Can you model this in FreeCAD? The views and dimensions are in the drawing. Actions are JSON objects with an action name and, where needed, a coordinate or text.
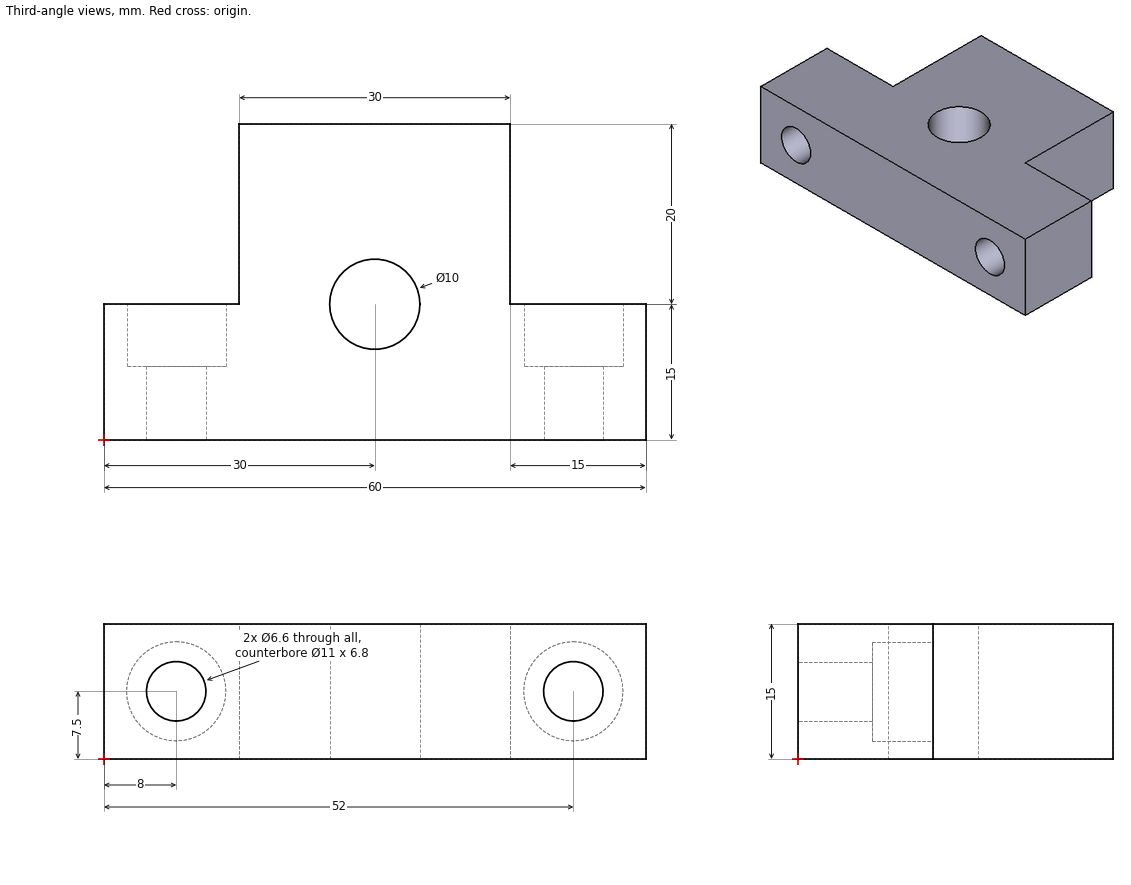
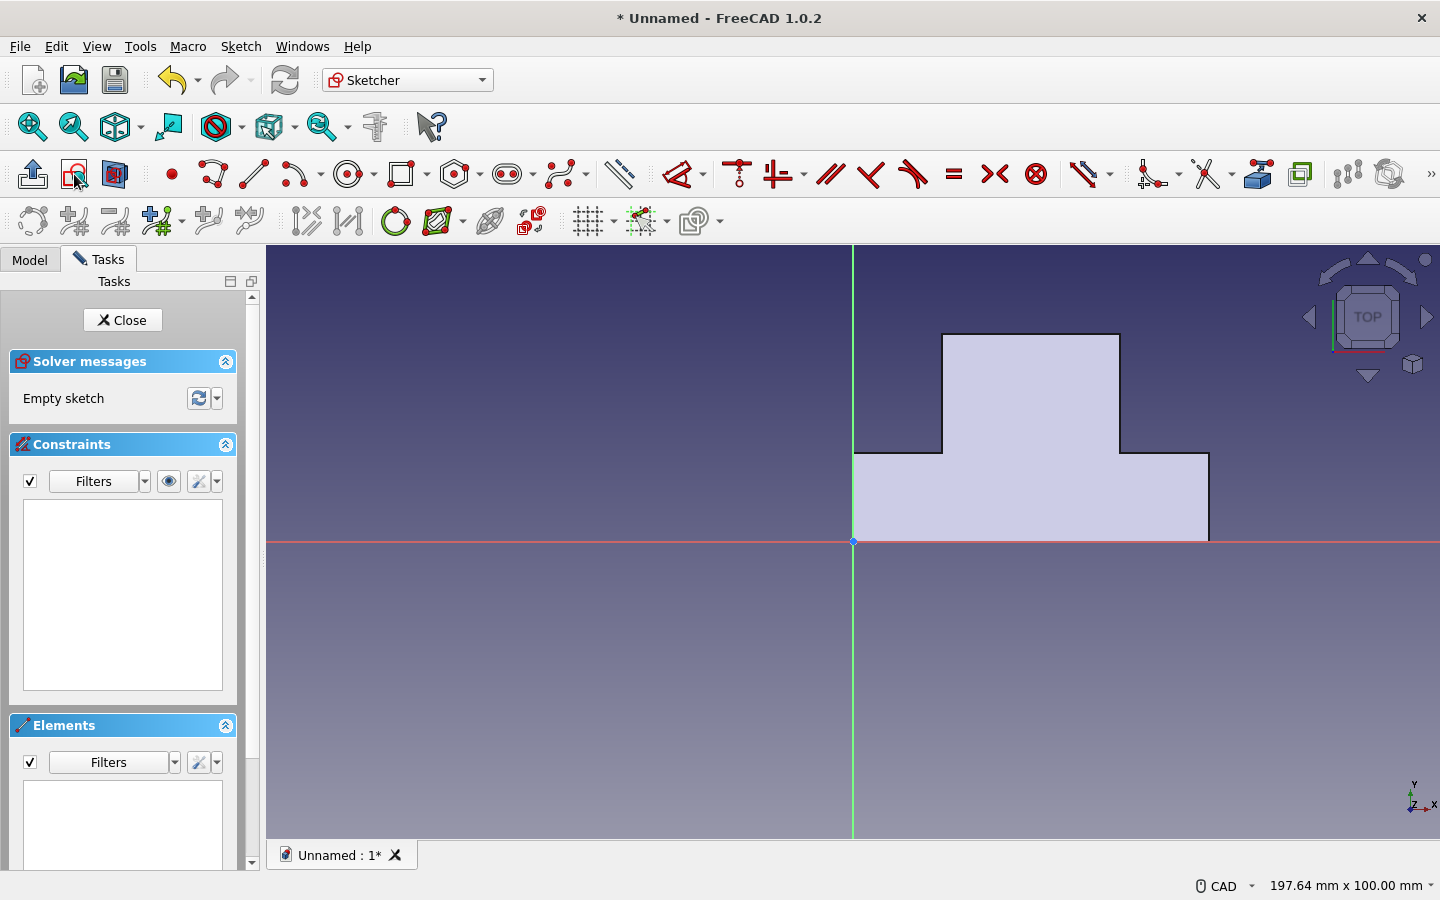
{"action": "scroll", "coordinate": [1080, 435], "scroll_direction": "up", "scroll_amount": 9}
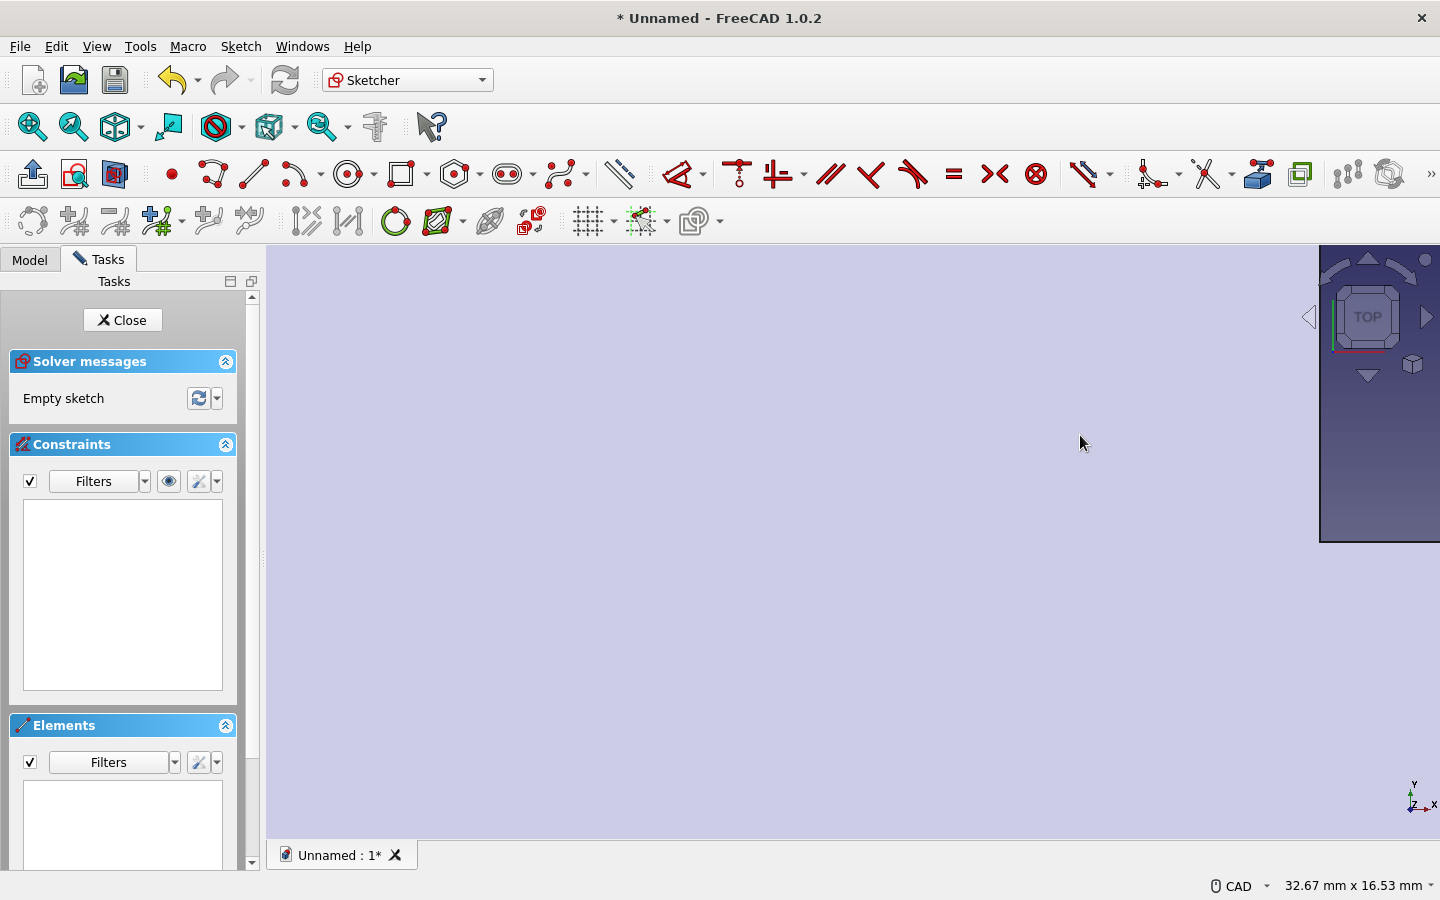
{"action": "left_click", "coordinate": [348, 174]}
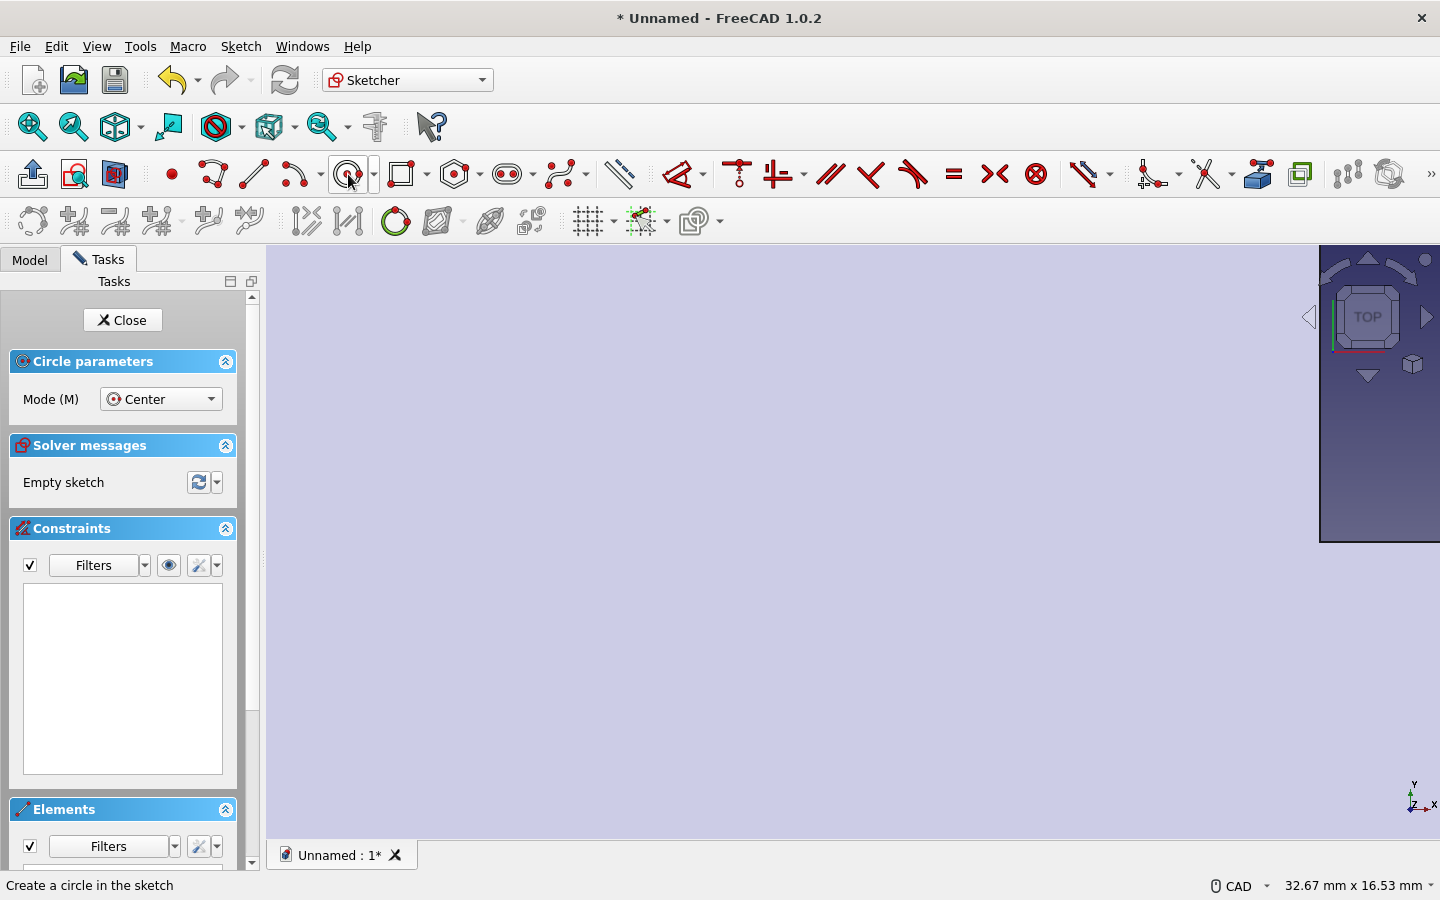
{"action": "left_click", "coordinate": [781, 542]}
{"action": "left_click", "coordinate": [908, 415]}
{"action": "key", "text": "Escape"}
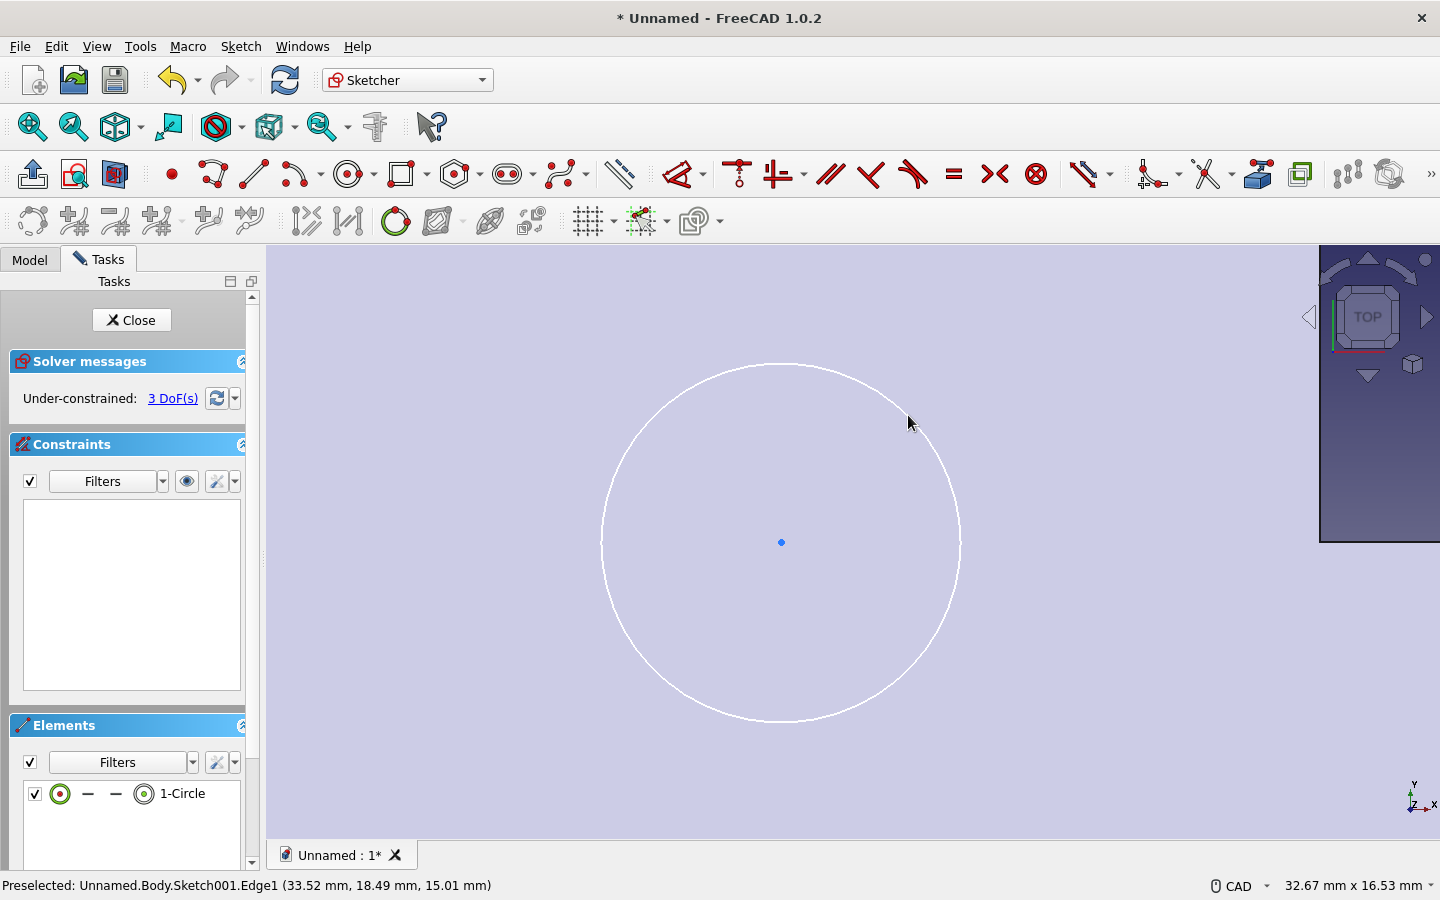
{"action": "left_click", "coordinate": [676, 174]}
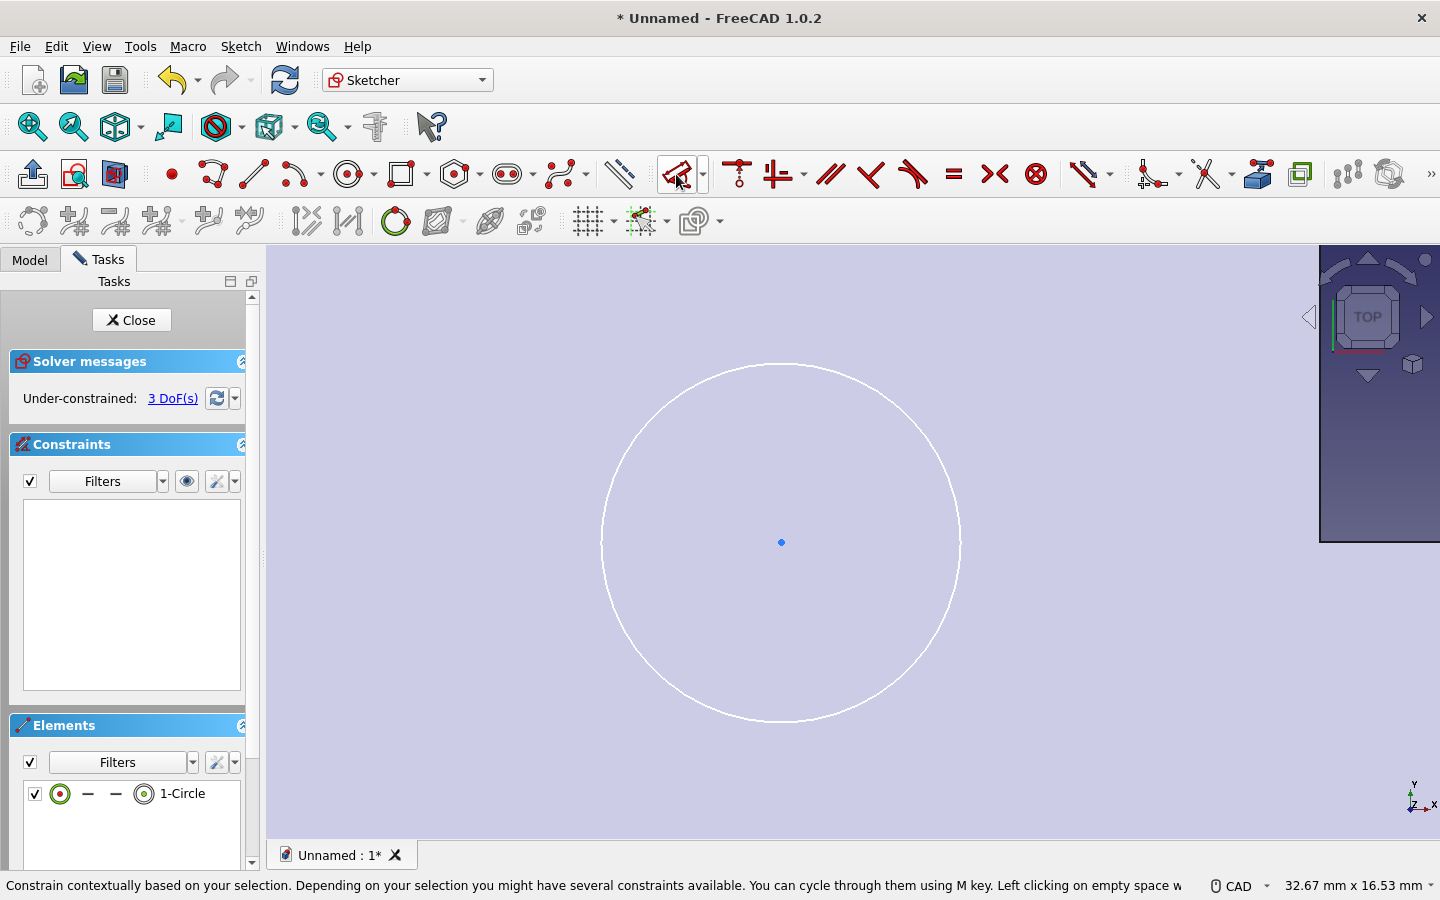
{"action": "left_click", "coordinate": [908, 416]}
{"action": "left_click", "coordinate": [931, 393]}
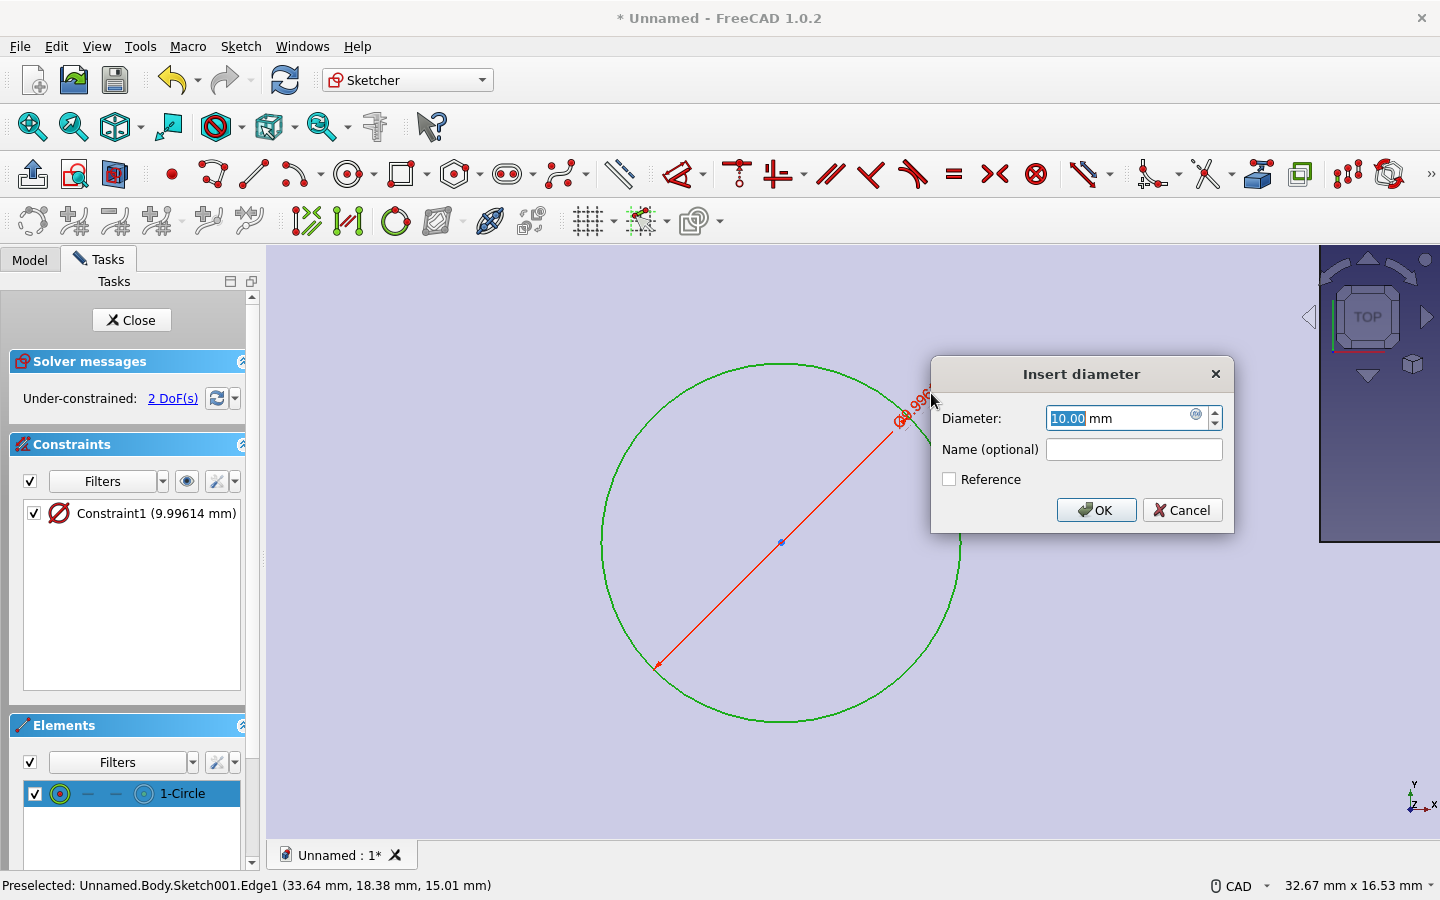
{"action": "type", "text": "10"}
{"action": "key", "text": "Return"}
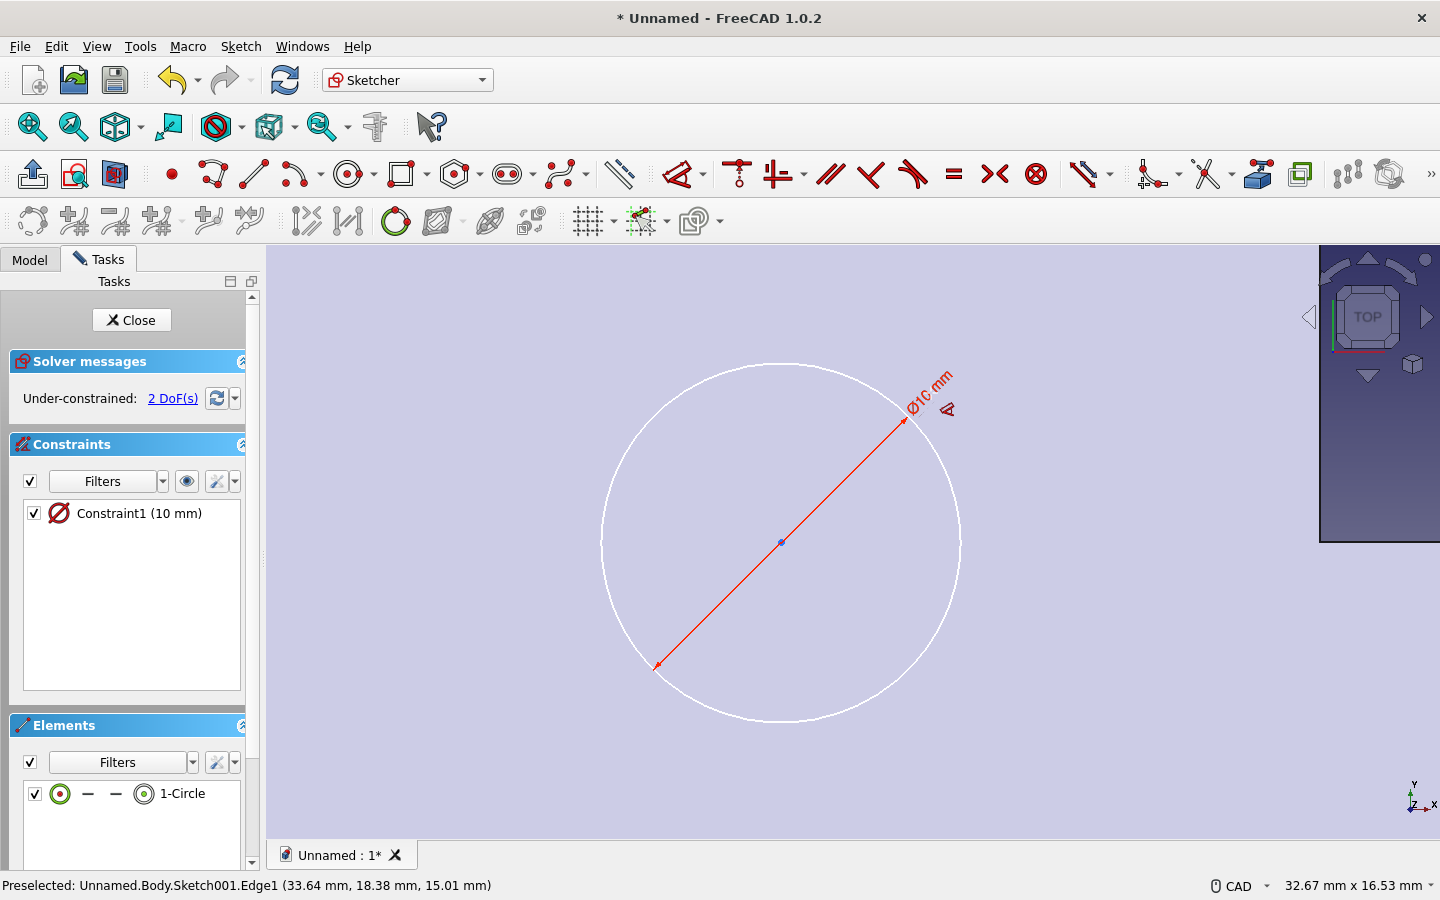
{"action": "left_click", "coordinate": [781, 543]}
{"action": "left_click", "coordinate": [537, 509]}